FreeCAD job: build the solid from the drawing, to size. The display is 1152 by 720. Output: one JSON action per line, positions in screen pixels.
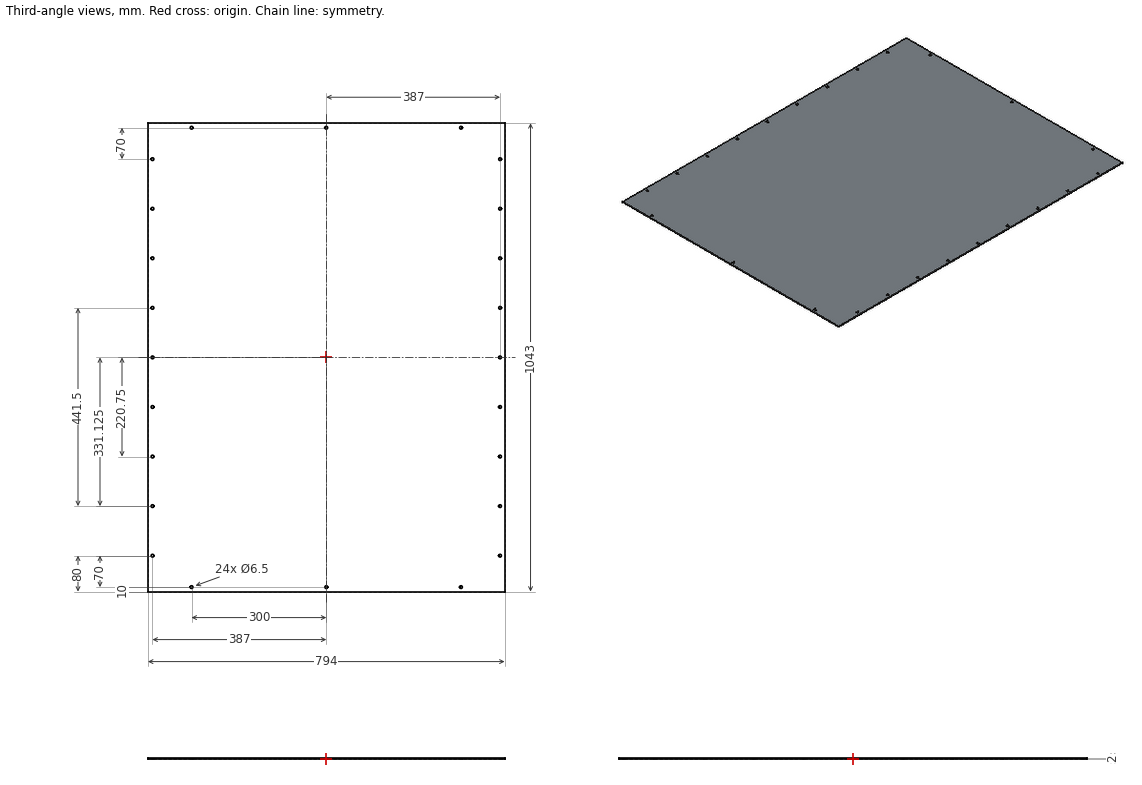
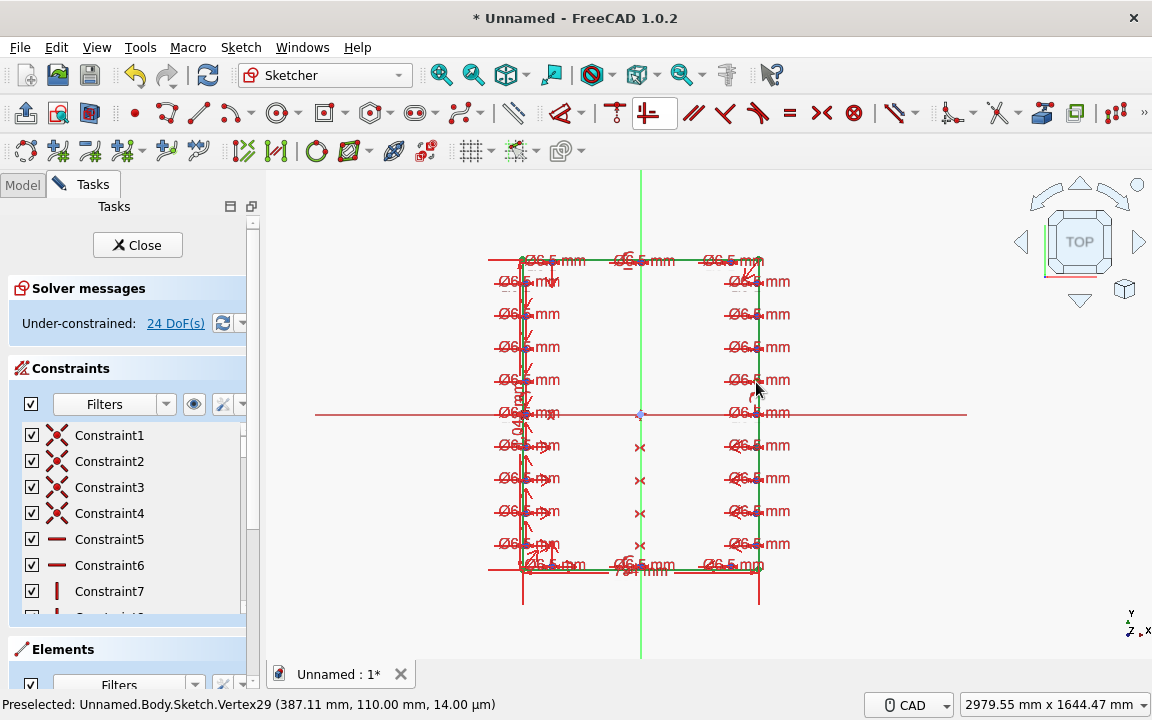
{"action": "left_click", "coordinate": [344, 415]}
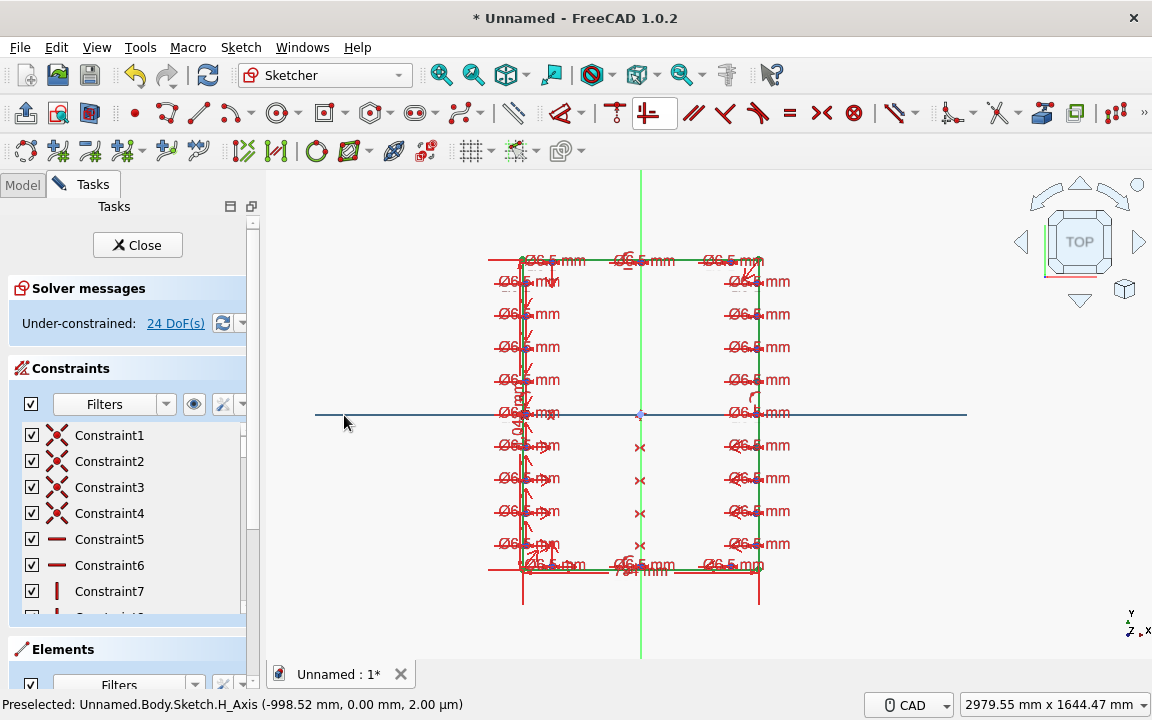
{"action": "left_click", "coordinate": [822, 114]}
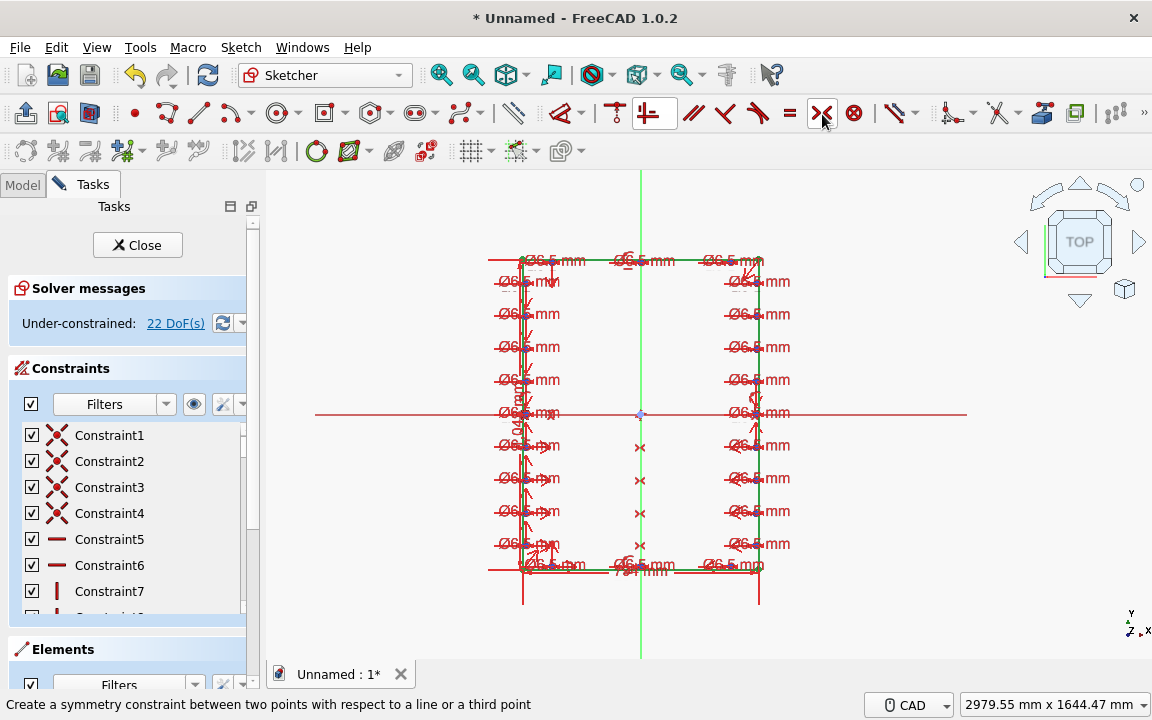
{"action": "left_click", "coordinate": [756, 480]}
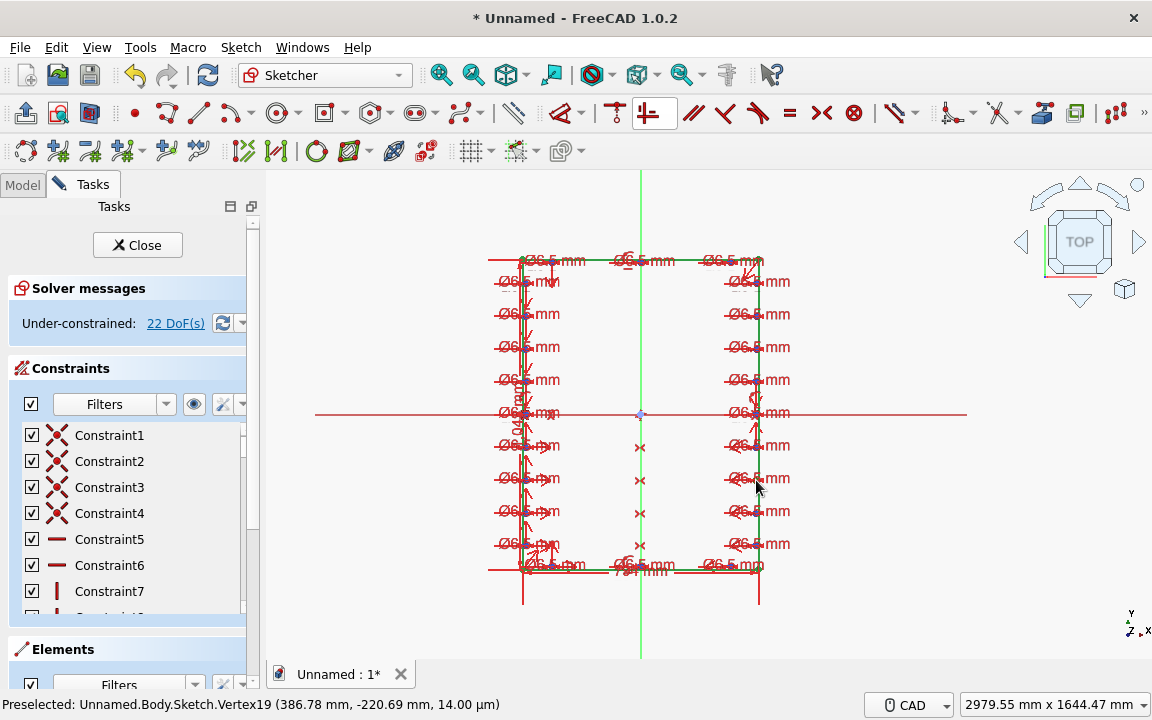
{"action": "left_click", "coordinate": [756, 349]}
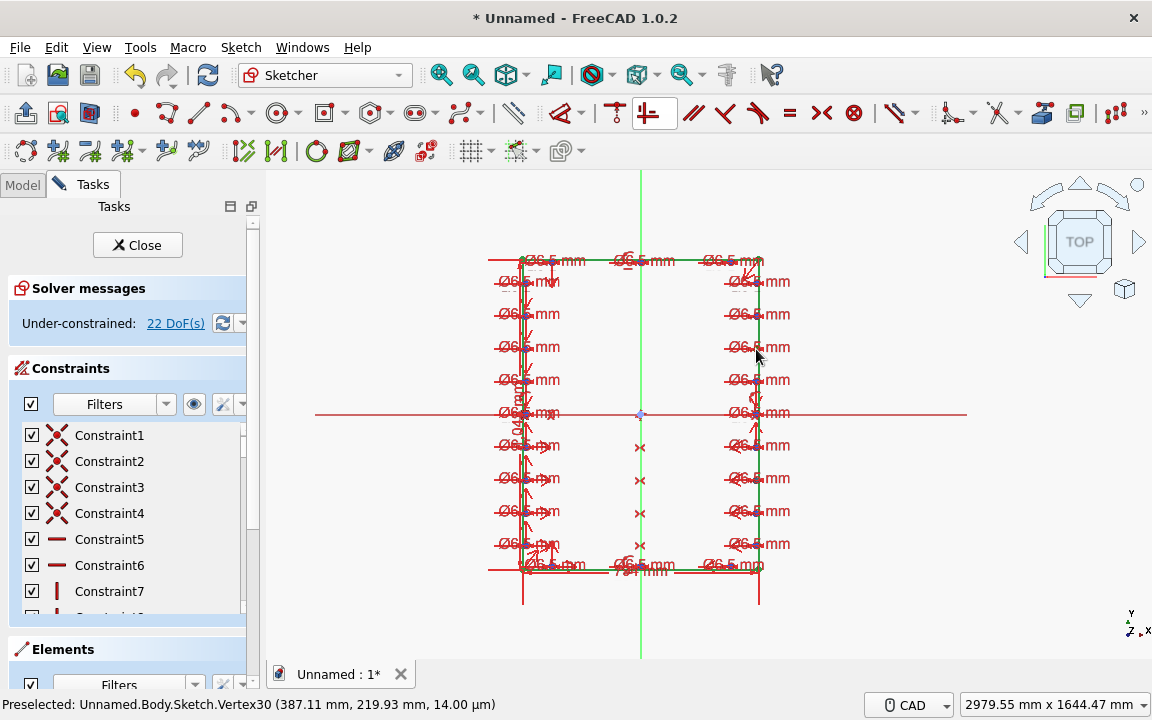
{"action": "left_click", "coordinate": [344, 415]}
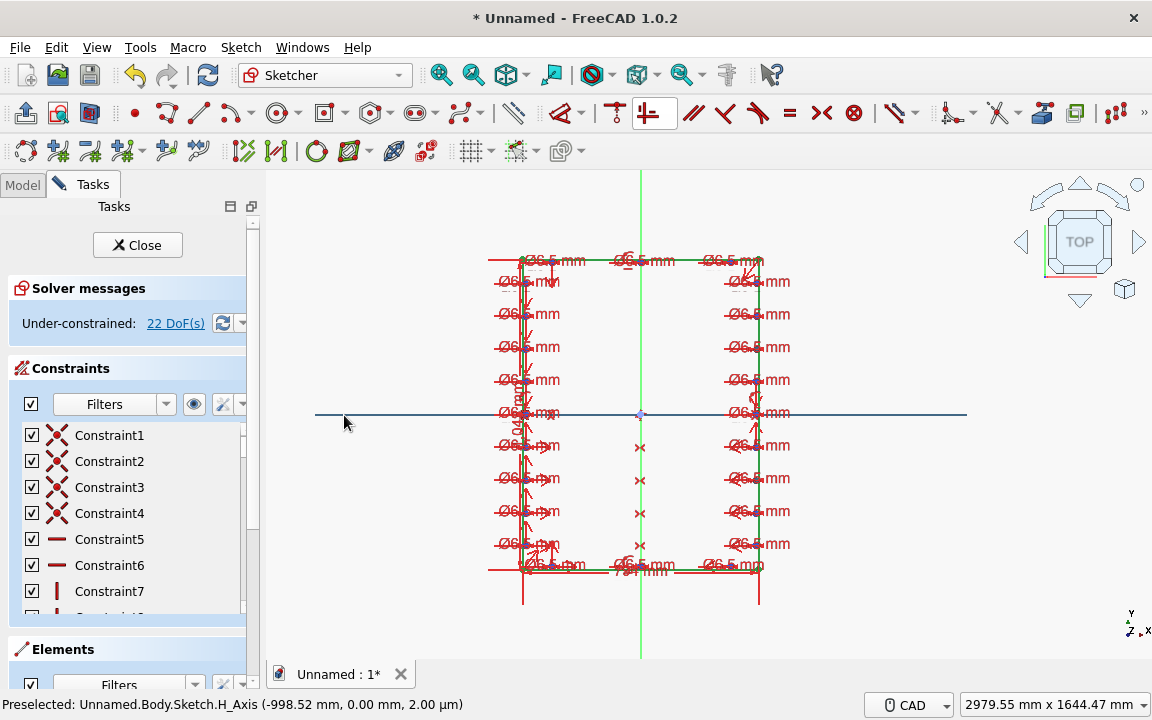
{"action": "left_click", "coordinate": [822, 114]}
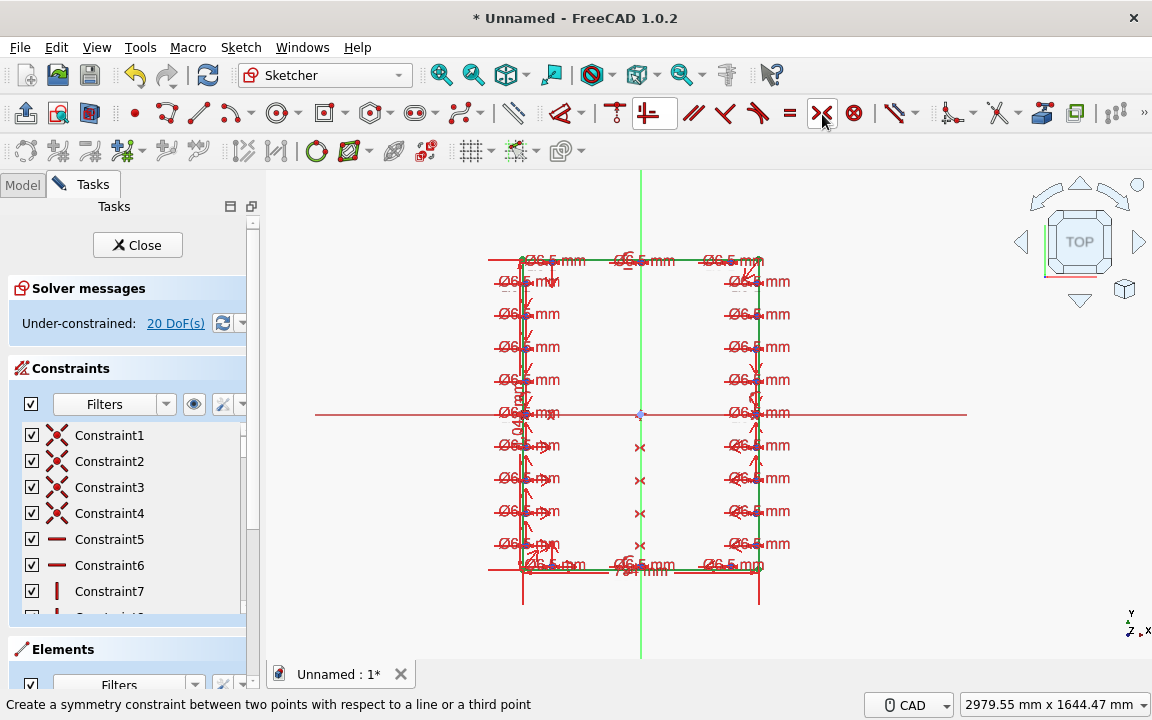
{"action": "left_click", "coordinate": [756, 513]}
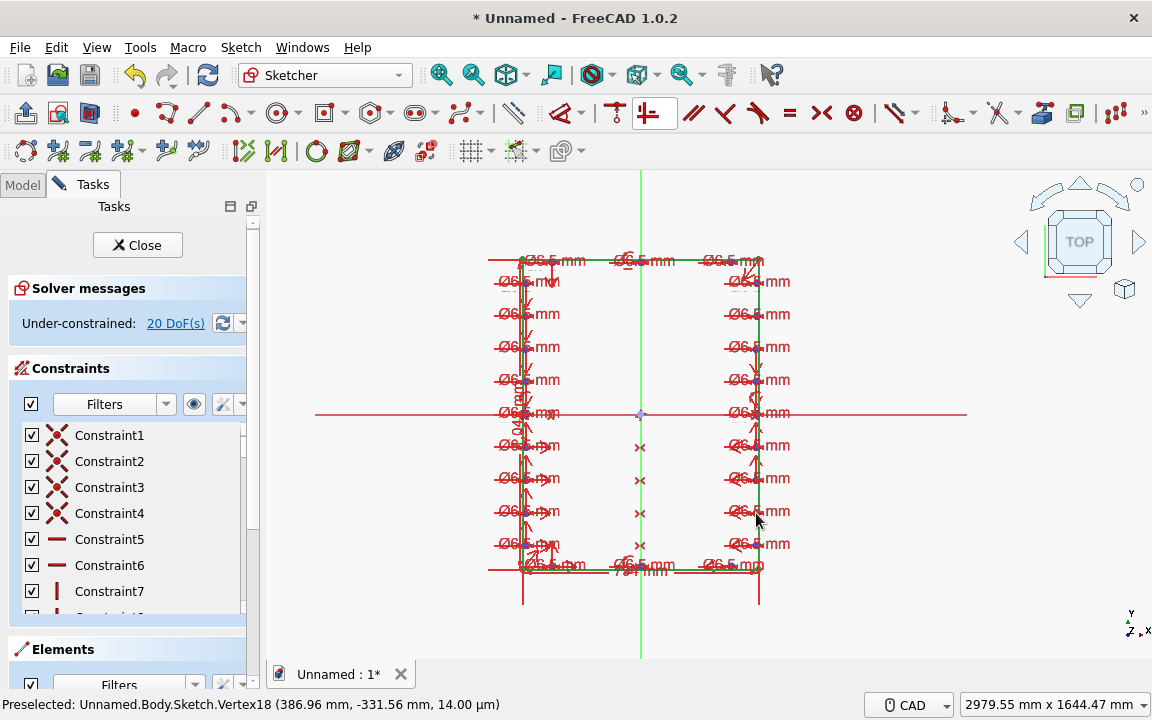
{"action": "left_click", "coordinate": [756, 316]}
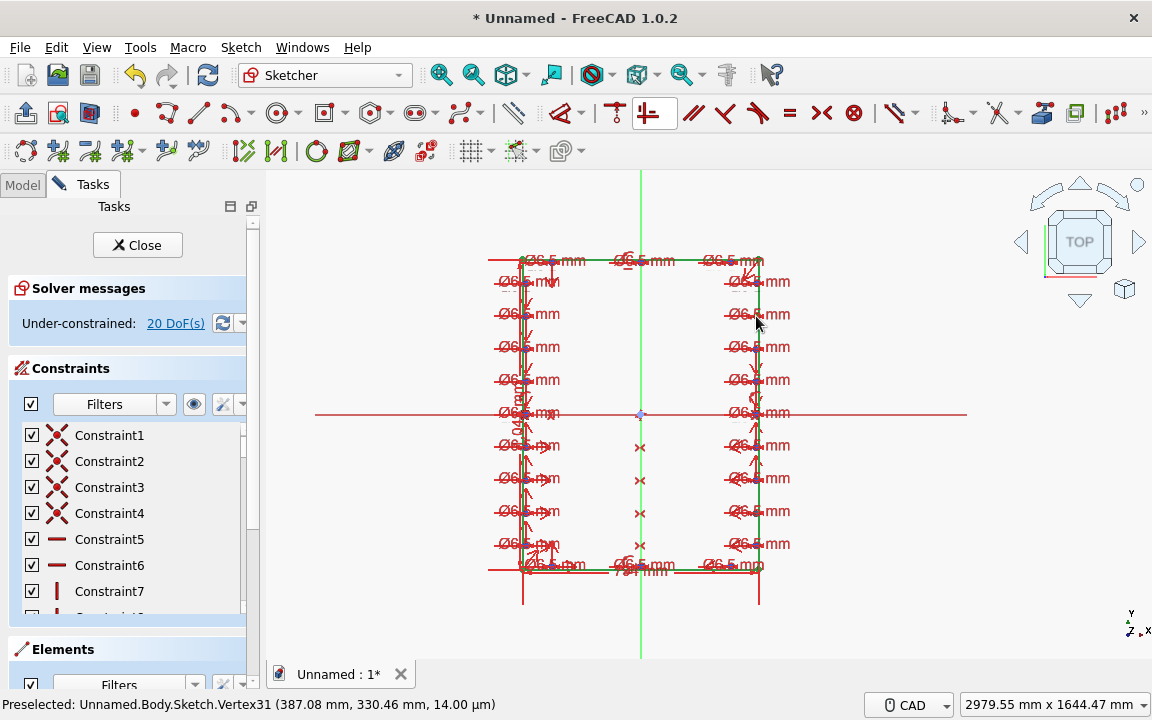
{"action": "left_click", "coordinate": [344, 415]}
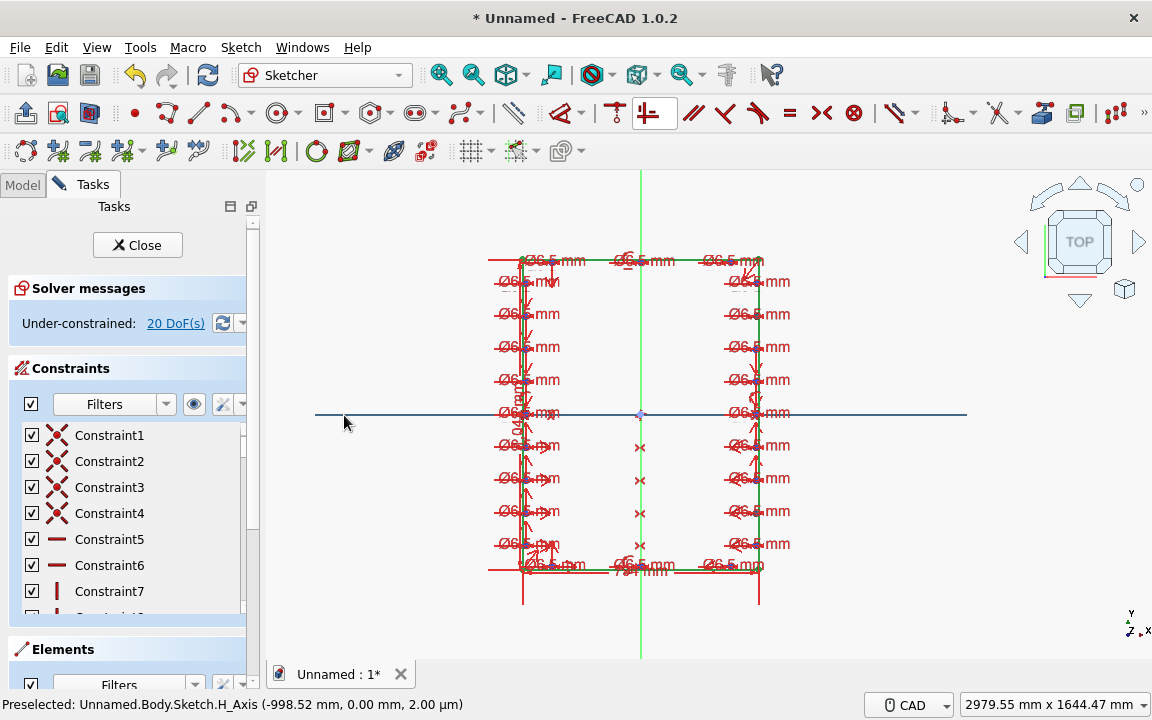
{"action": "left_click", "coordinate": [822, 114]}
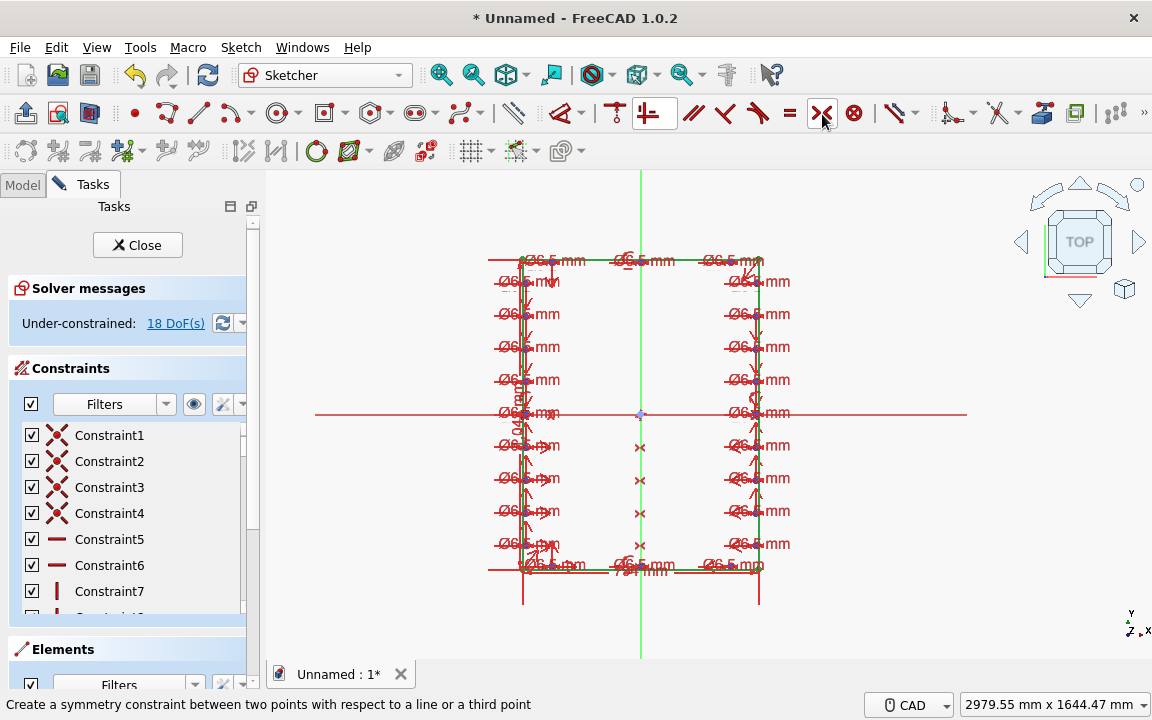
{"action": "left_click", "coordinate": [756, 546]}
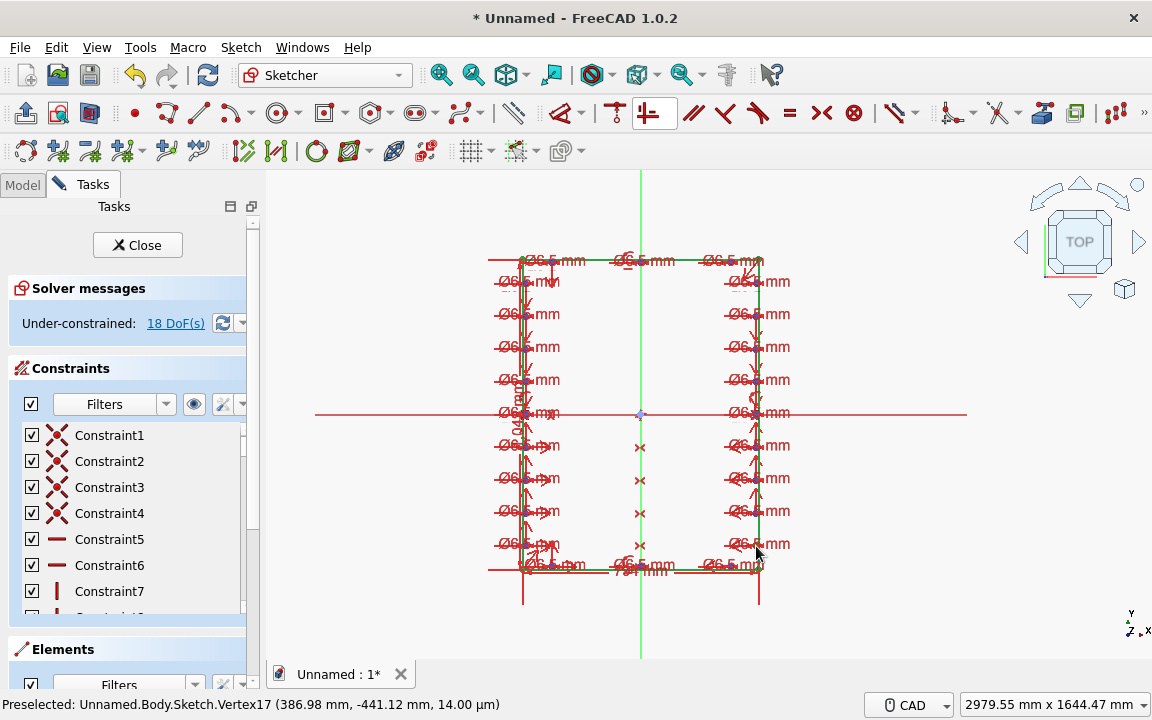
{"action": "left_click", "coordinate": [756, 284]}